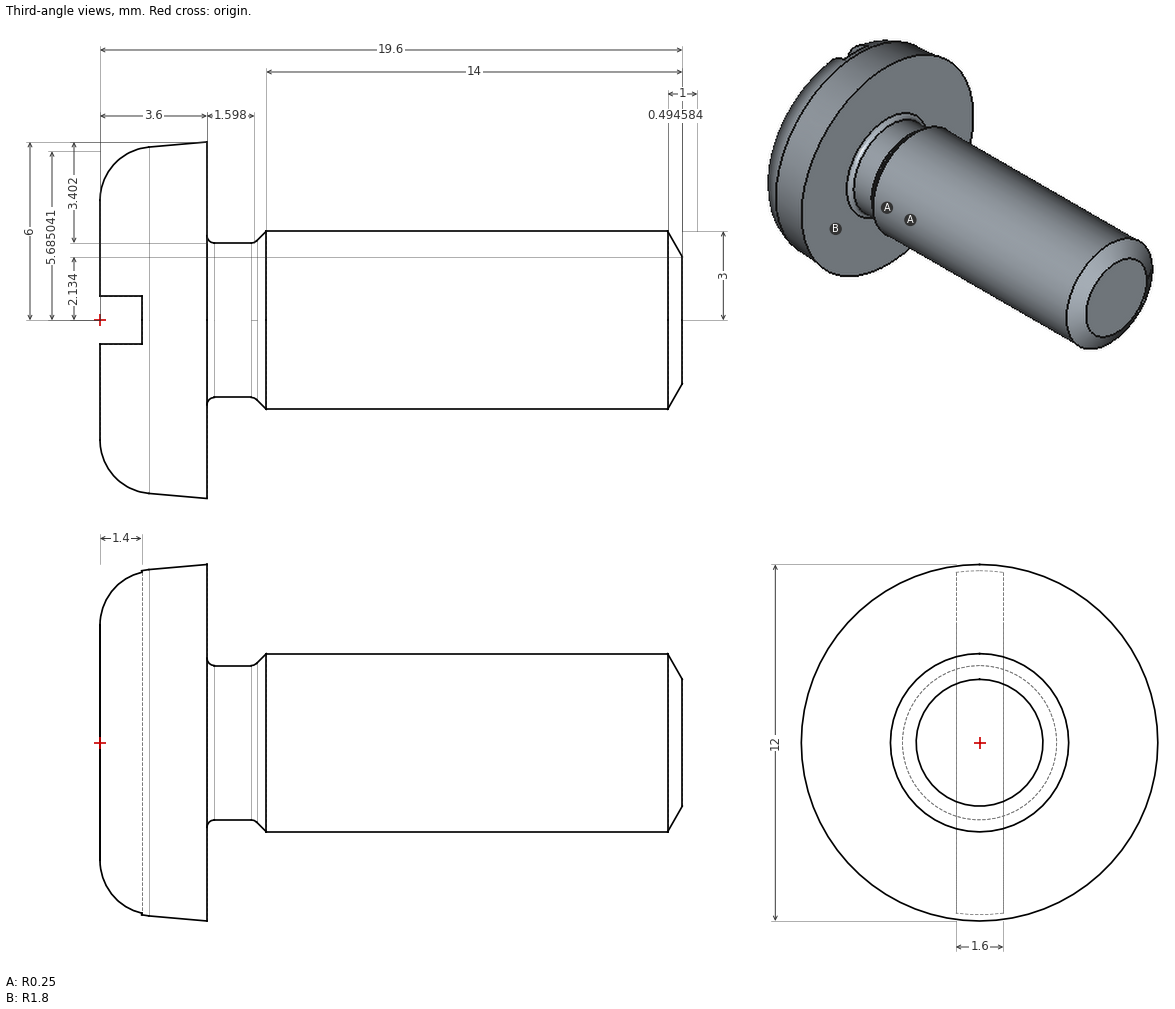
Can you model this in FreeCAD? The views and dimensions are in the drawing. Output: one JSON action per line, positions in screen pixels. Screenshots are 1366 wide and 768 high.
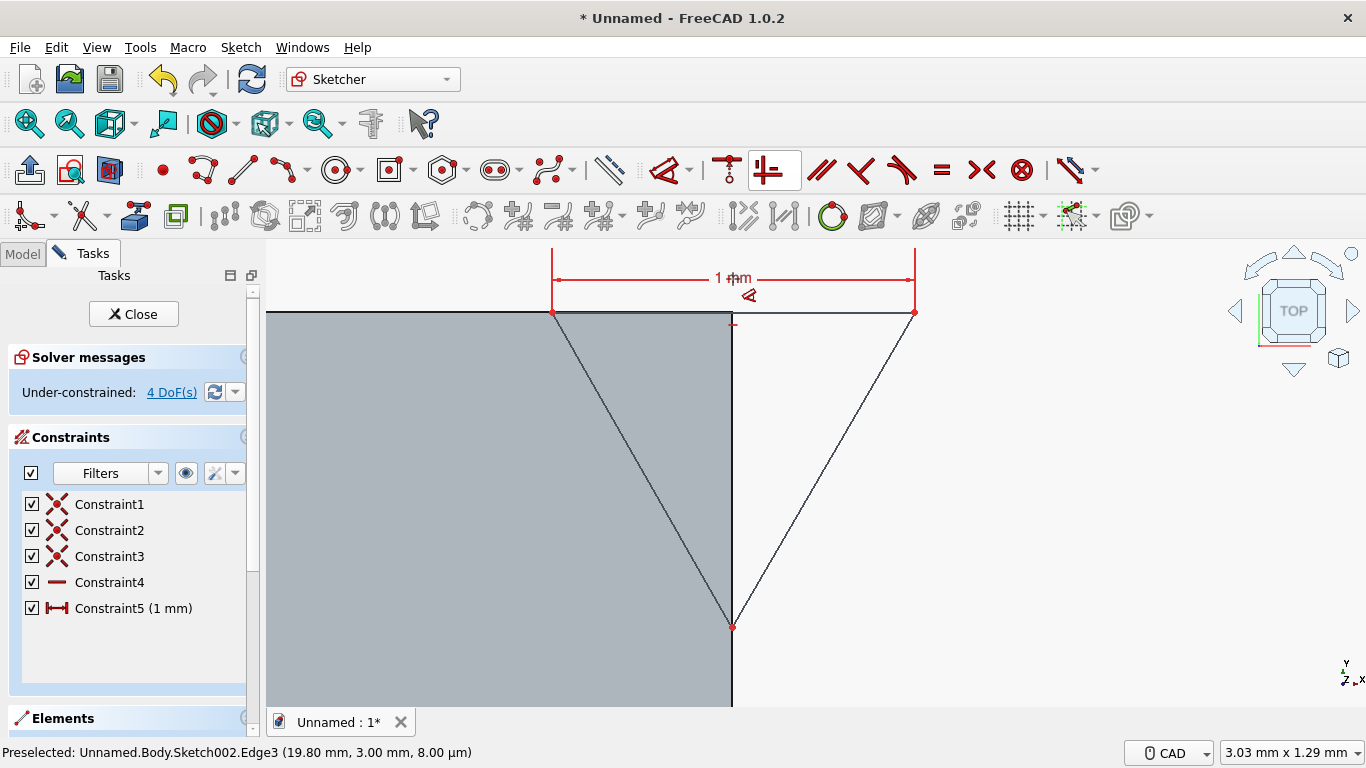
{"action": "left_click", "coordinate": [552, 313]}
{"action": "left_click", "coordinate": [586, 496]}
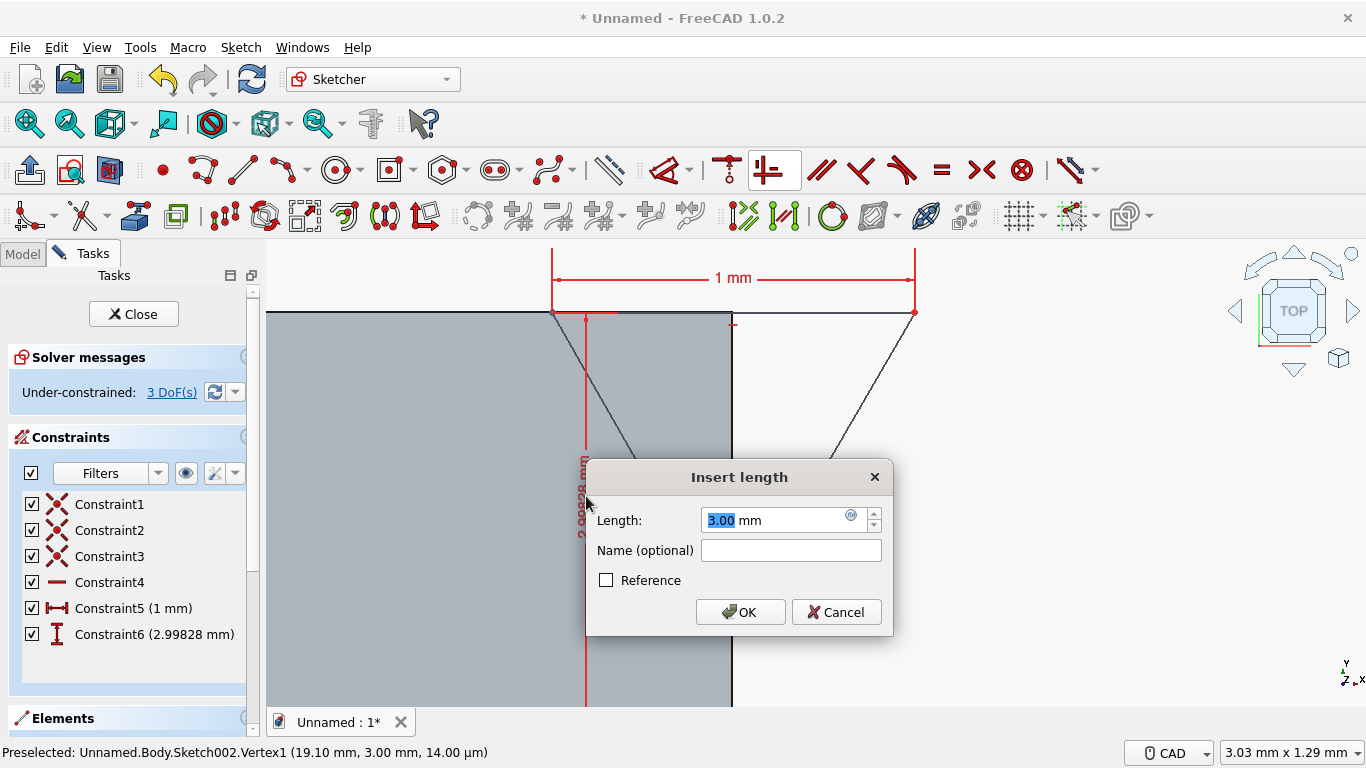
{"action": "type", "text": "3"}
{"action": "key", "text": "Return"}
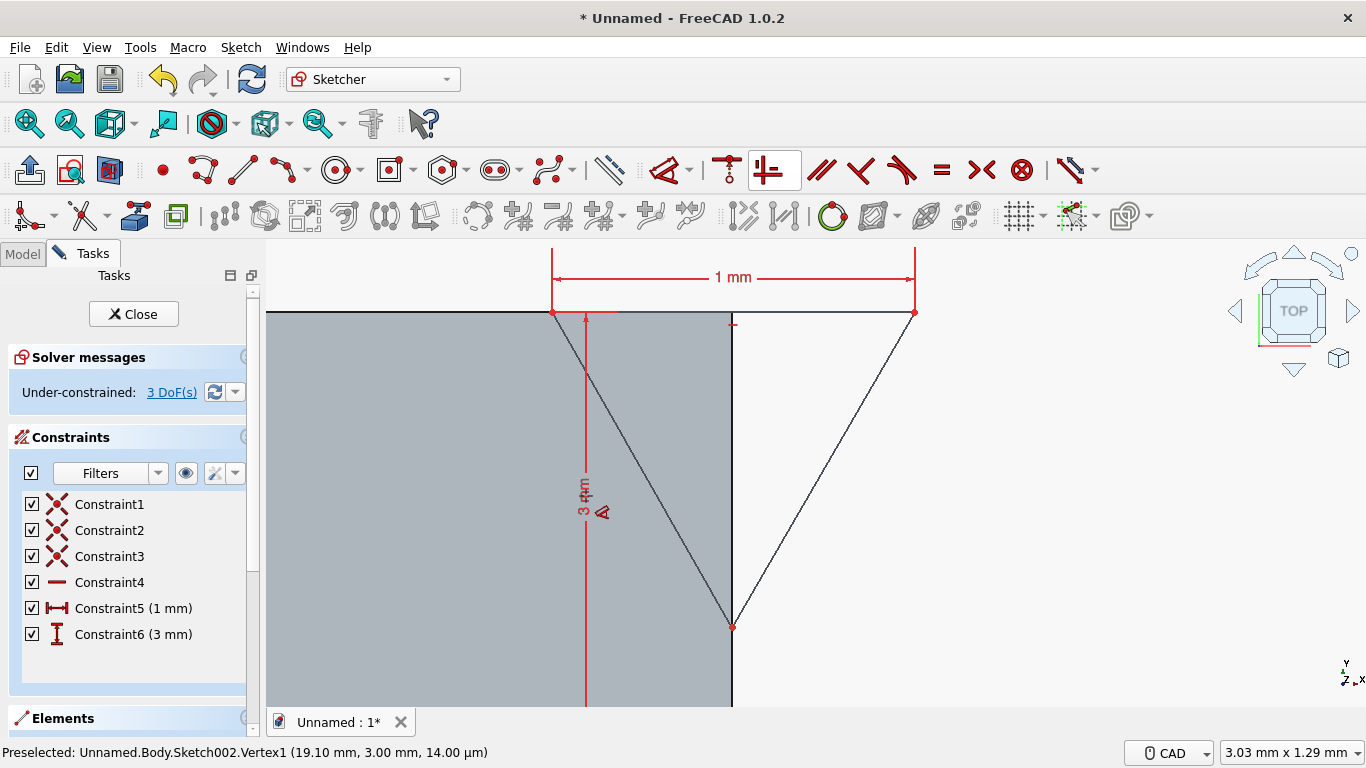
{"action": "left_click", "coordinate": [732, 628]}
{"action": "left_click", "coordinate": [513, 594]}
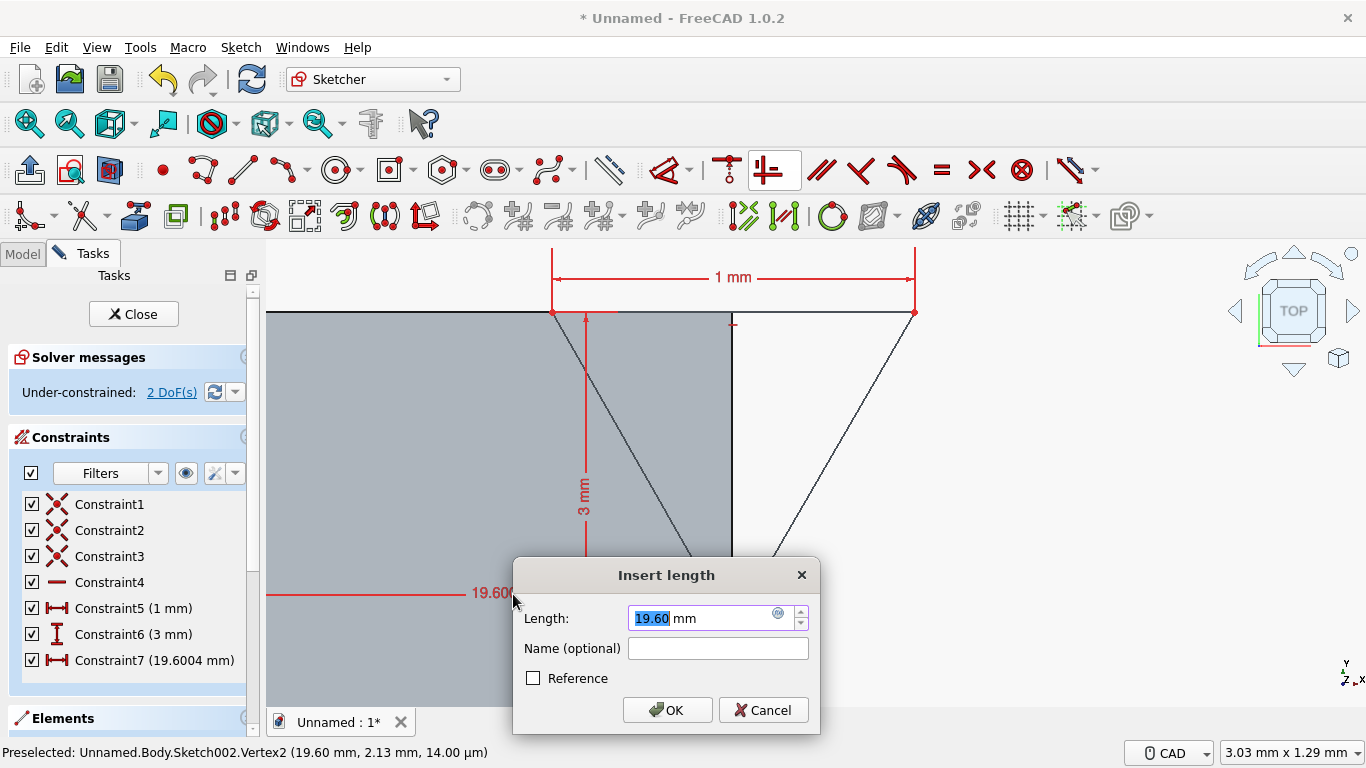
{"action": "type", "text": "19.6"}
{"action": "key", "text": "Return"}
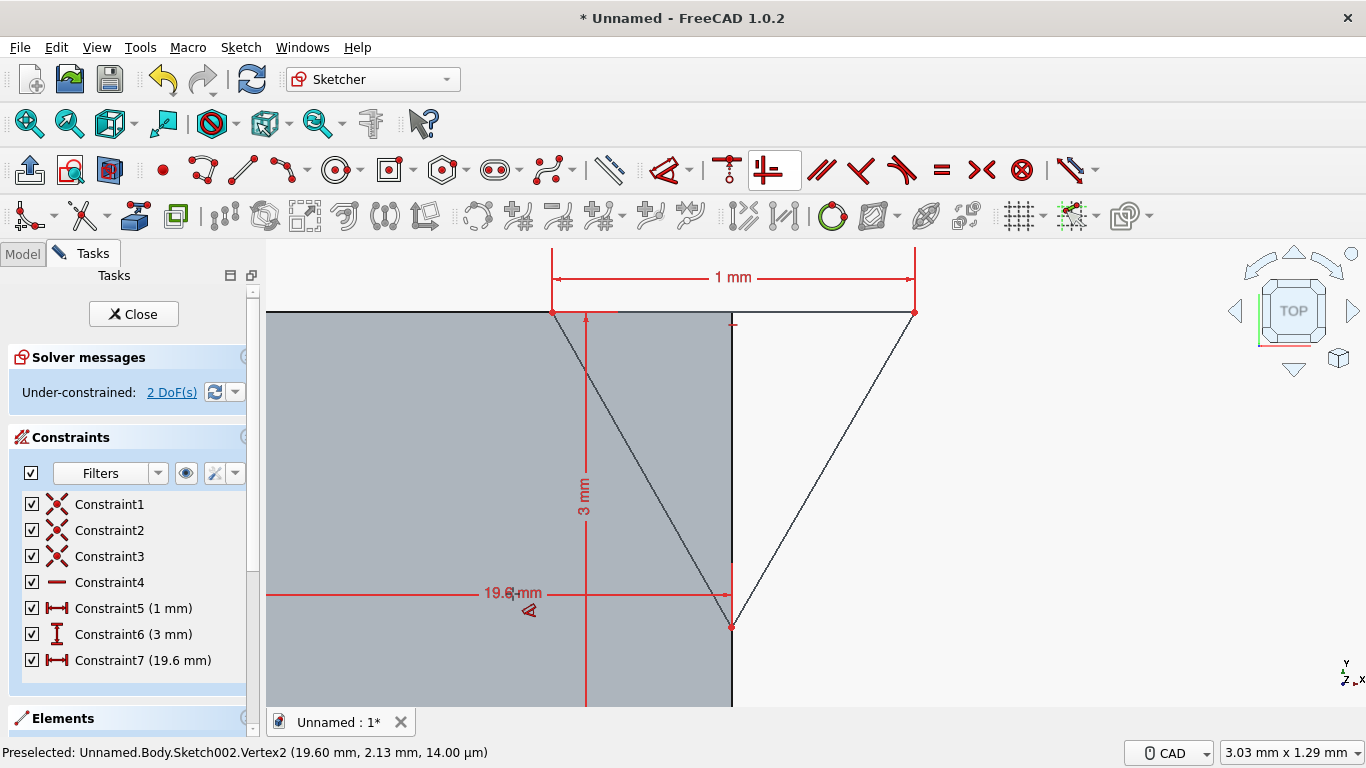
{"action": "left_click", "coordinate": [732, 628]}
{"action": "left_click", "coordinate": [766, 653]}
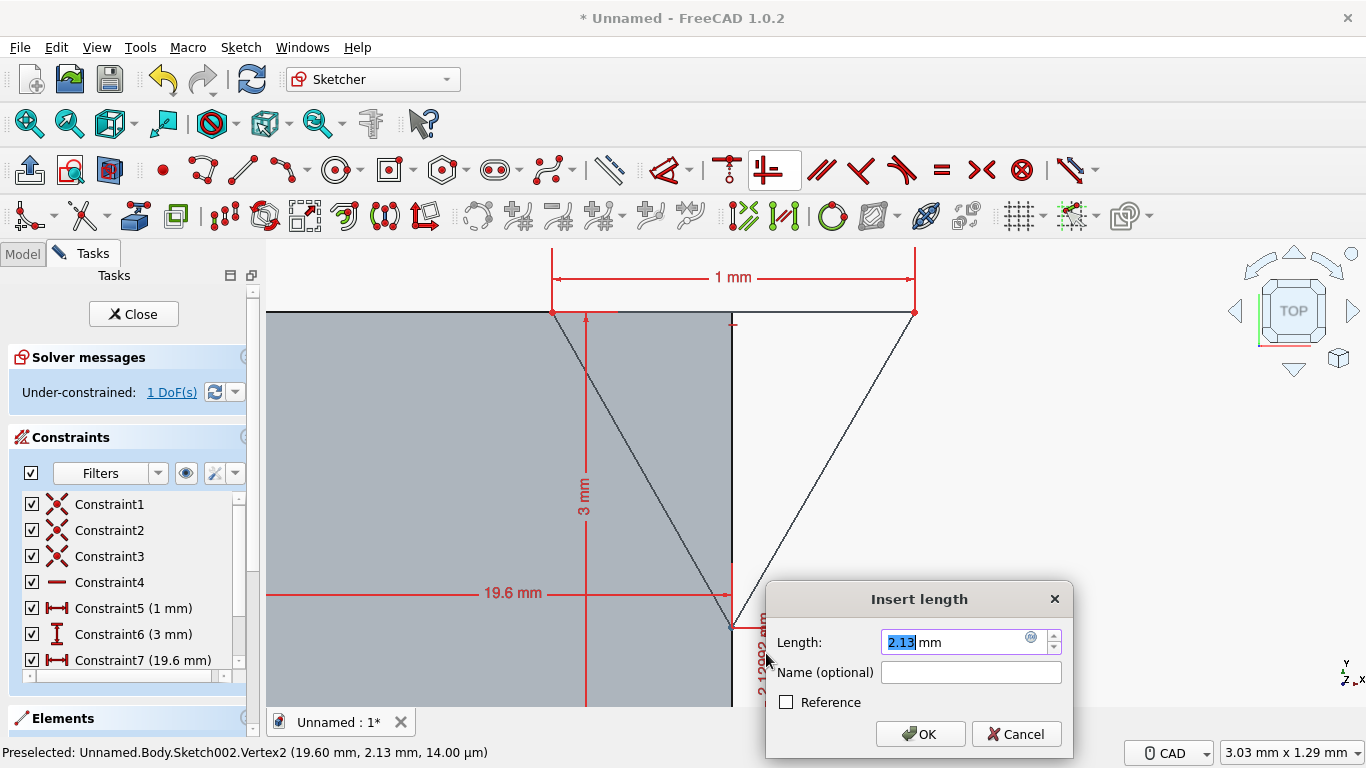
{"action": "type", "text": "2.134"}
{"action": "key", "text": "Return"}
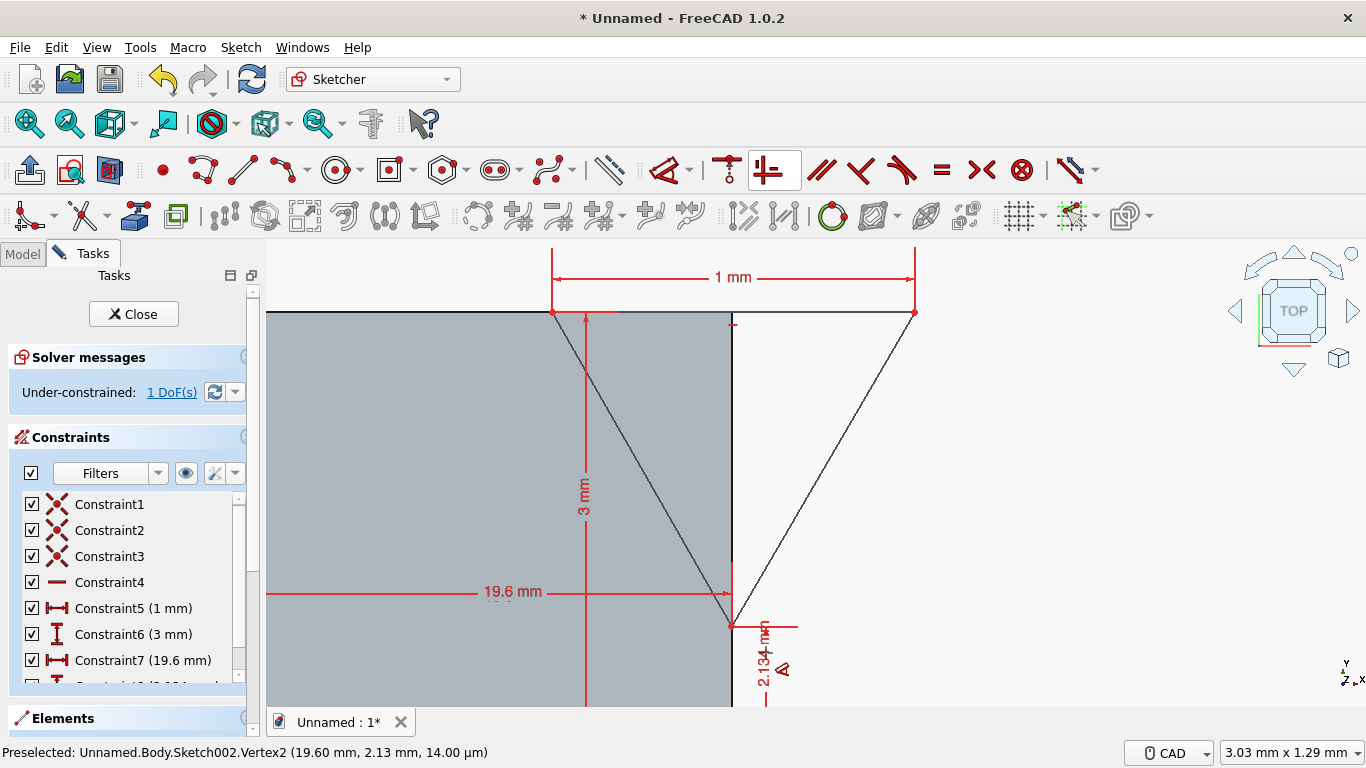
{"action": "left_click", "coordinate": [606, 407]}
{"action": "left_click", "coordinate": [642, 661]}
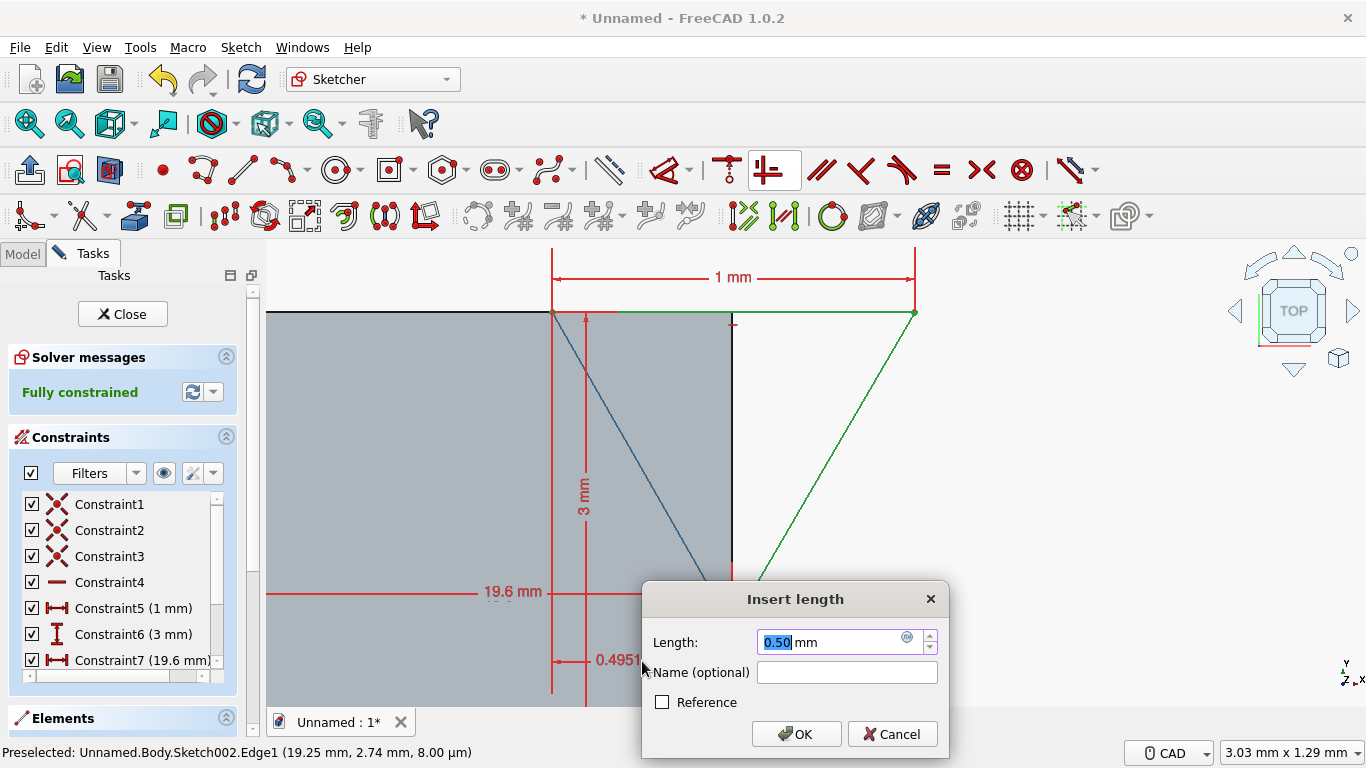
{"action": "type", "text": "0.494584"}
{"action": "key", "text": "Return"}
{"action": "key", "text": "Escape"}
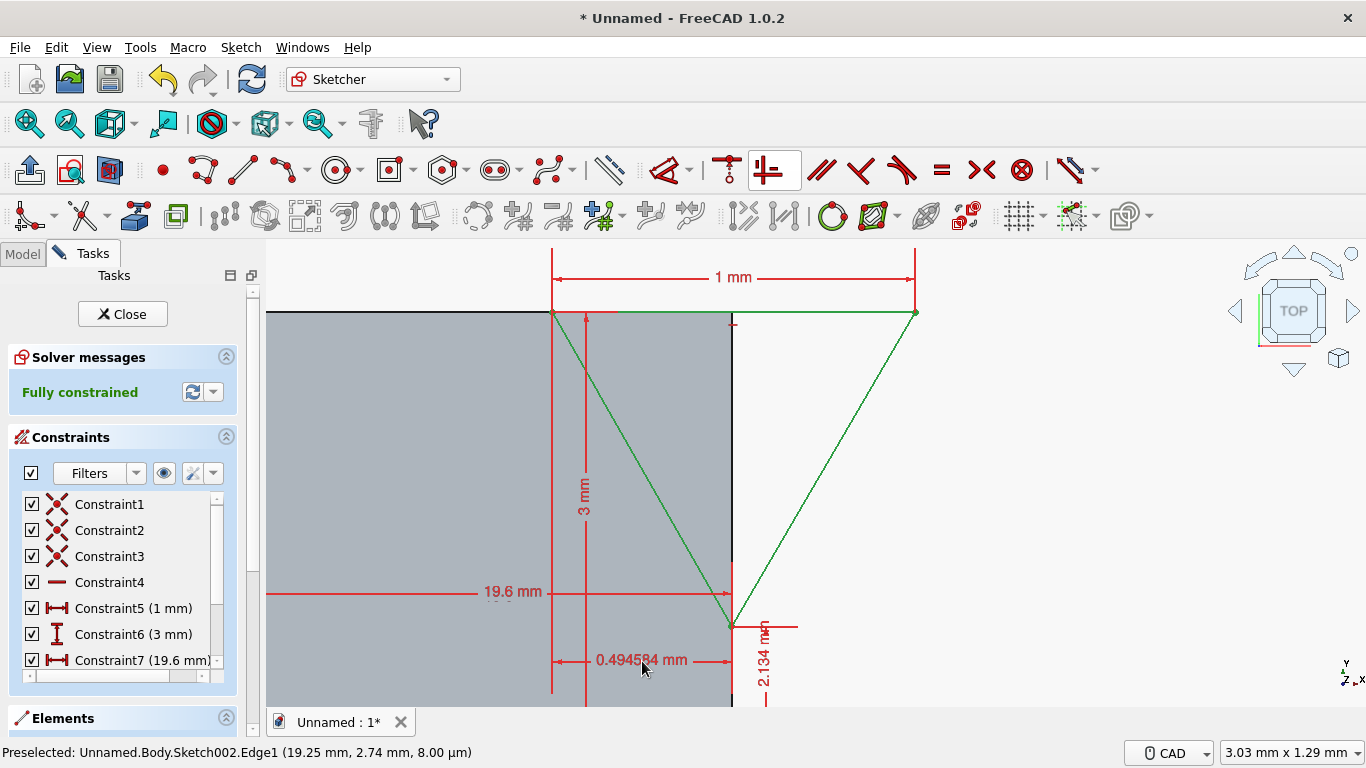
{"action": "left_click", "coordinate": [123, 314]}